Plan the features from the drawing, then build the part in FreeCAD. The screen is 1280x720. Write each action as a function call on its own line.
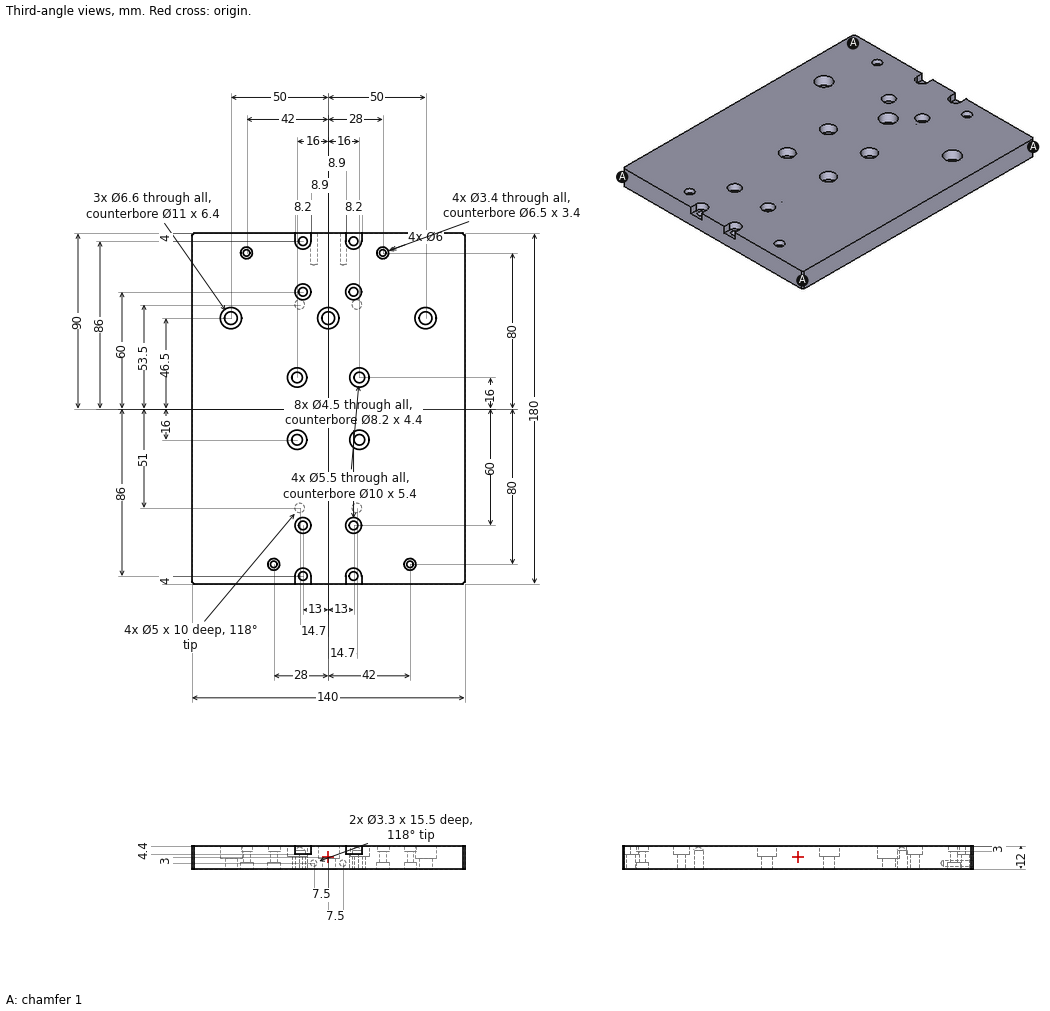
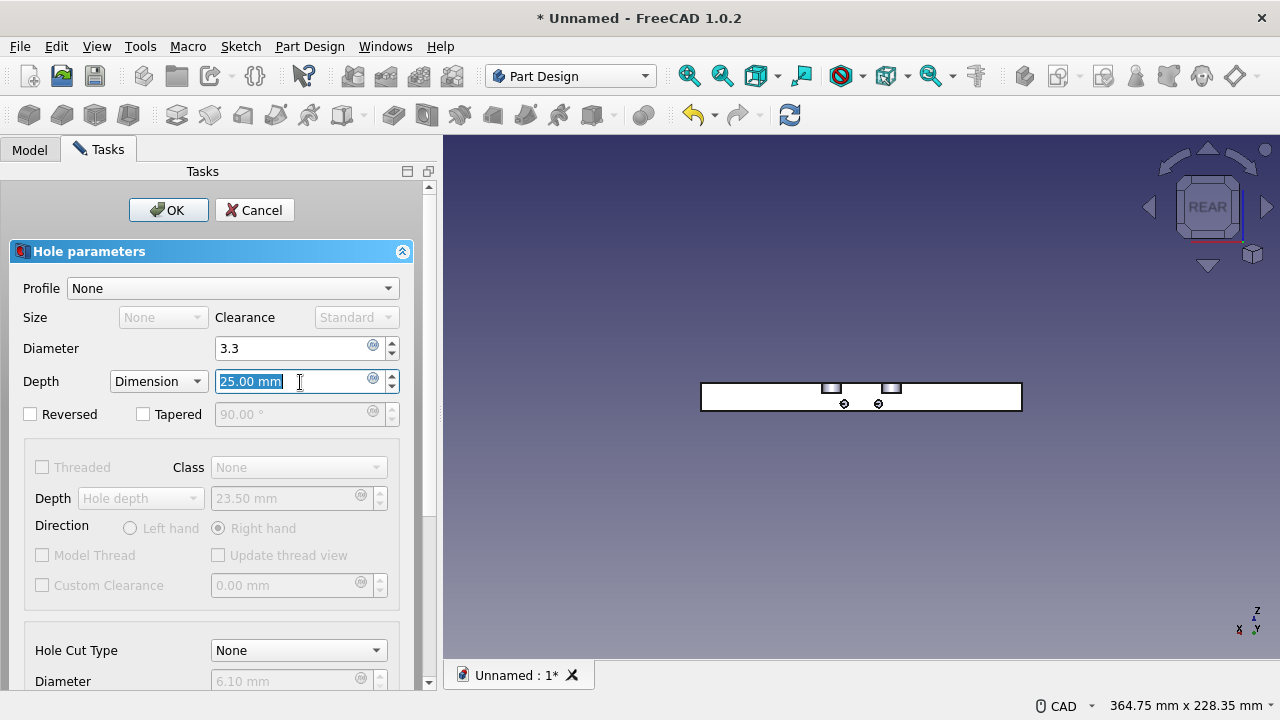
text(15.5)
key(Tab)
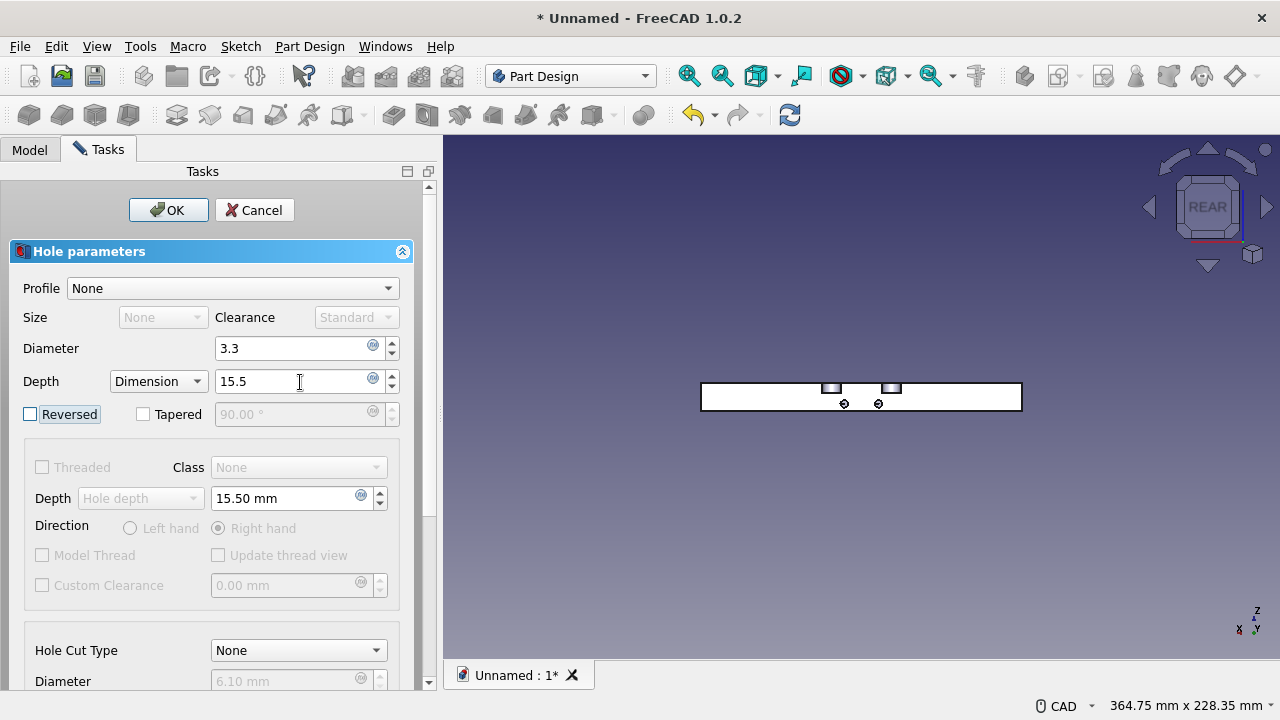
click(169, 210)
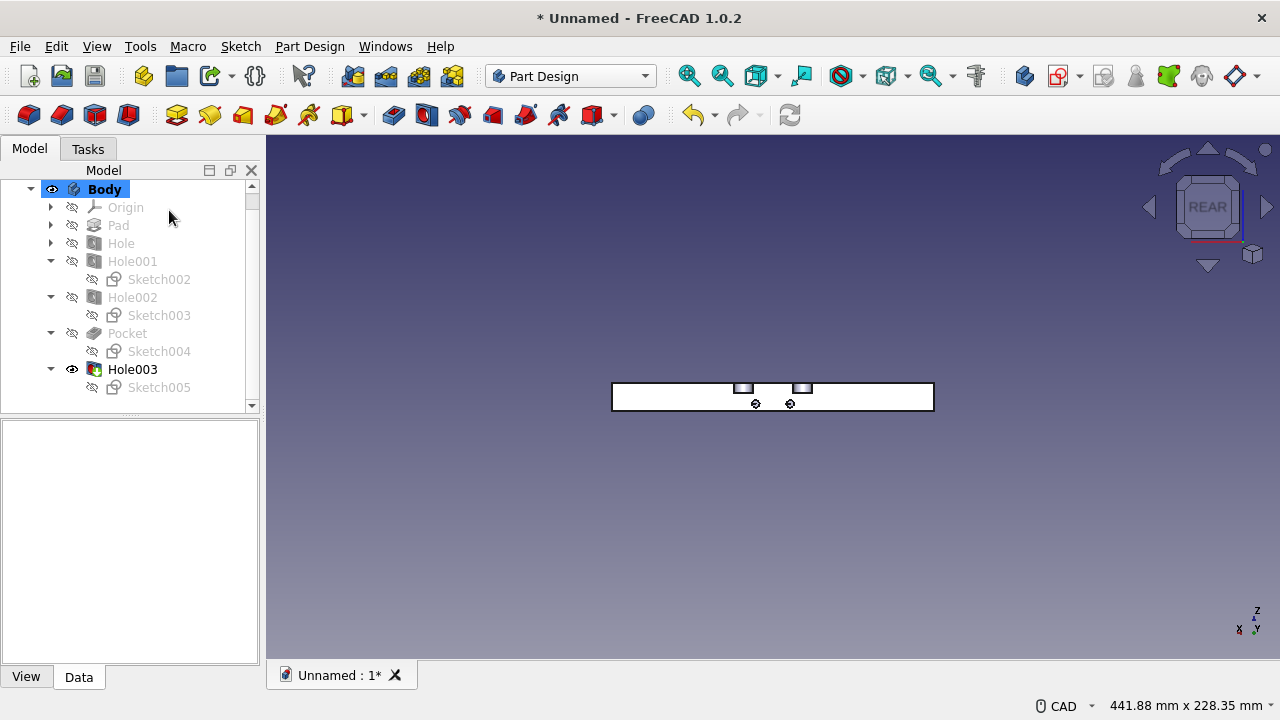
click(690, 76)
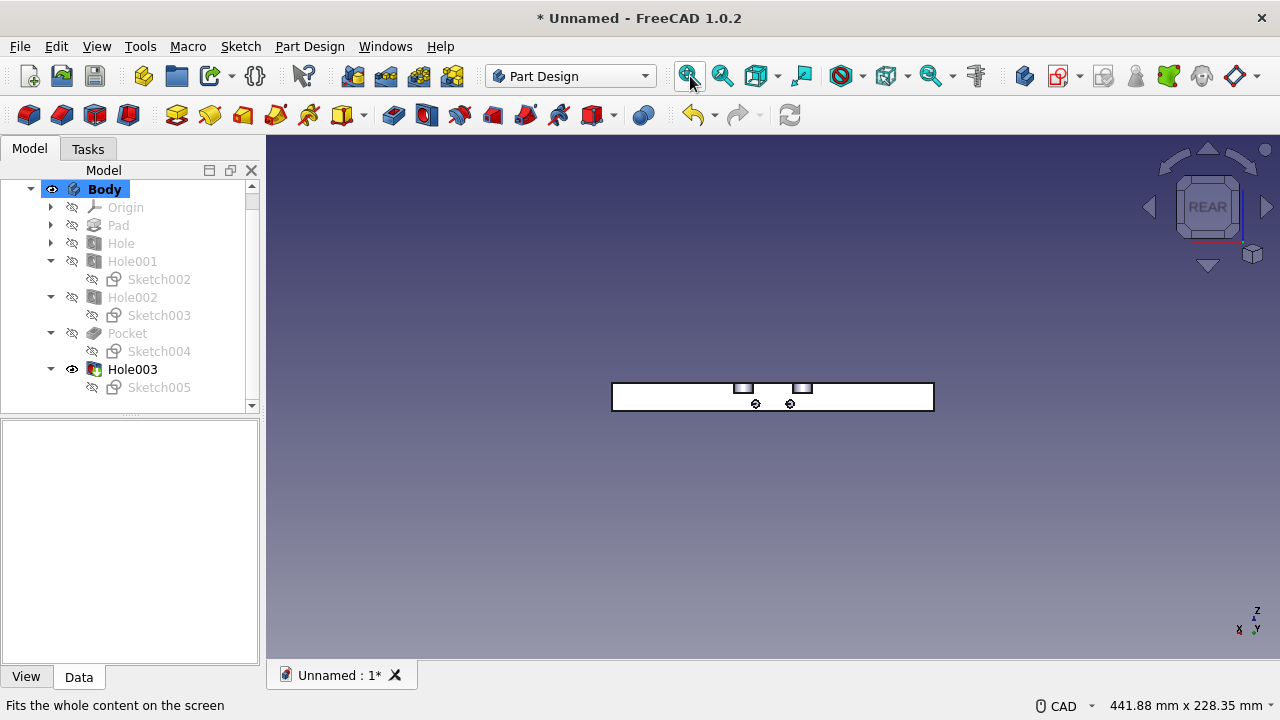
key(0)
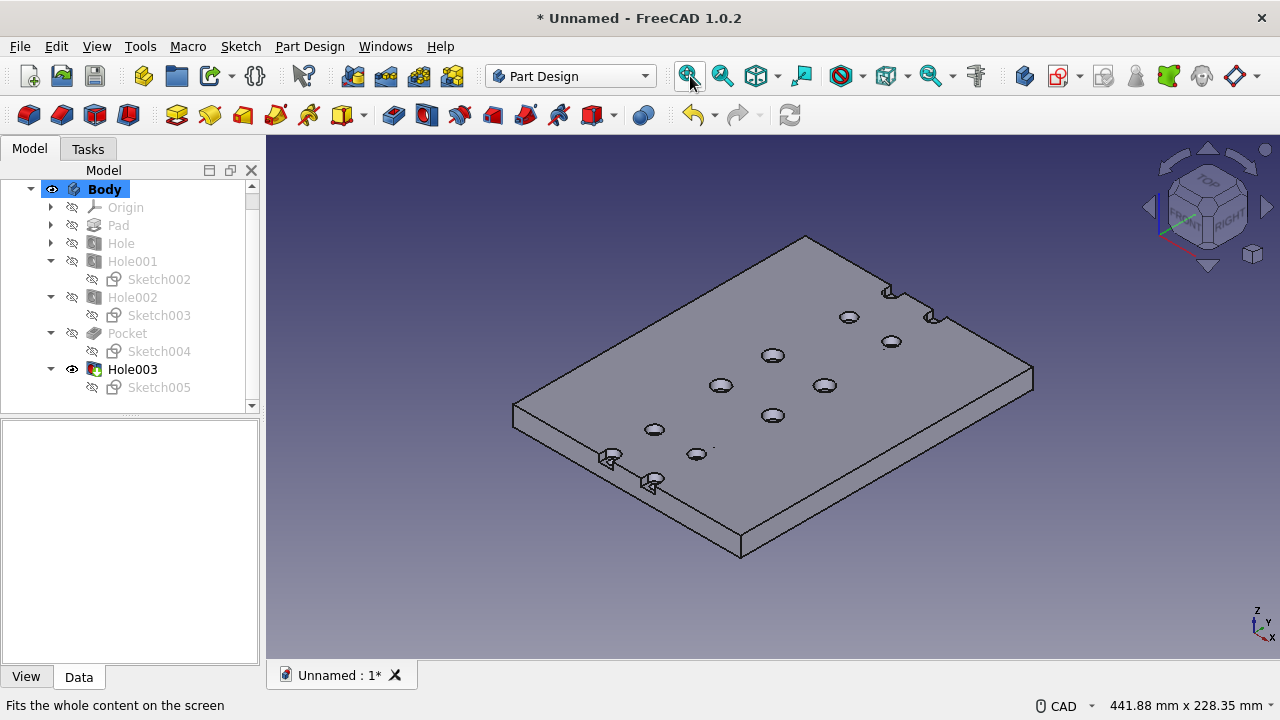
click(921, 374)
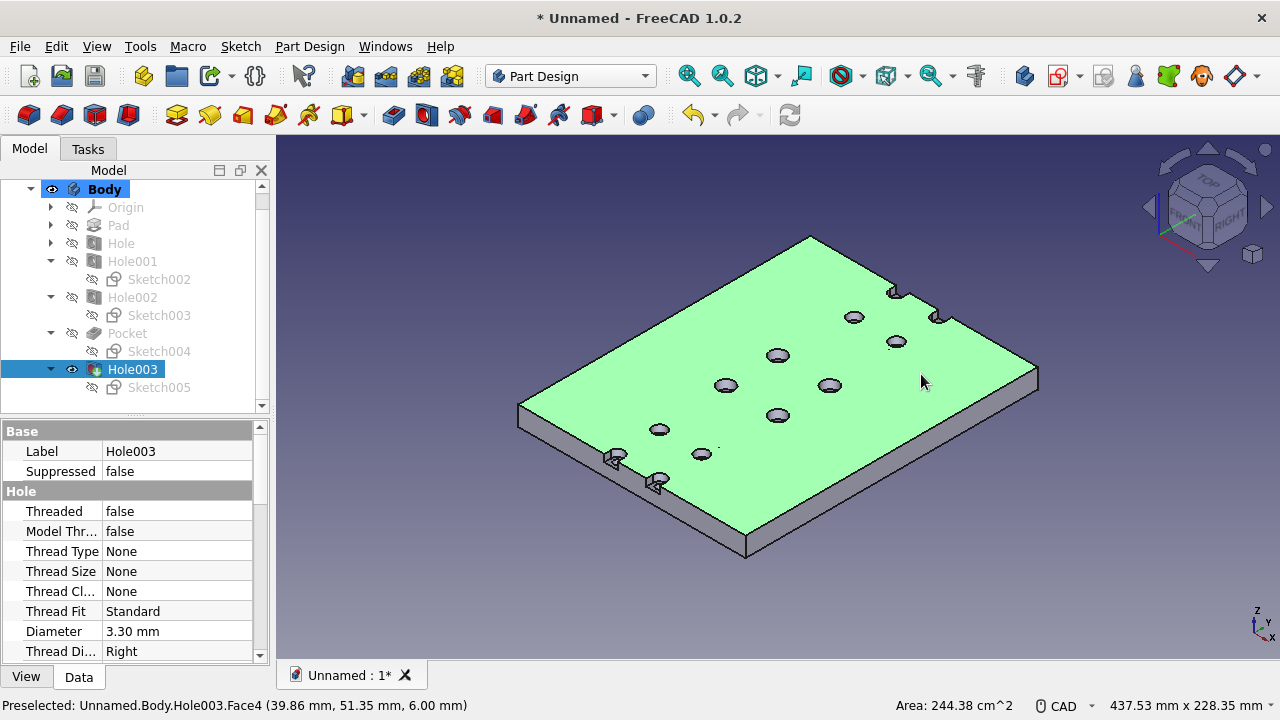
click(1058, 76)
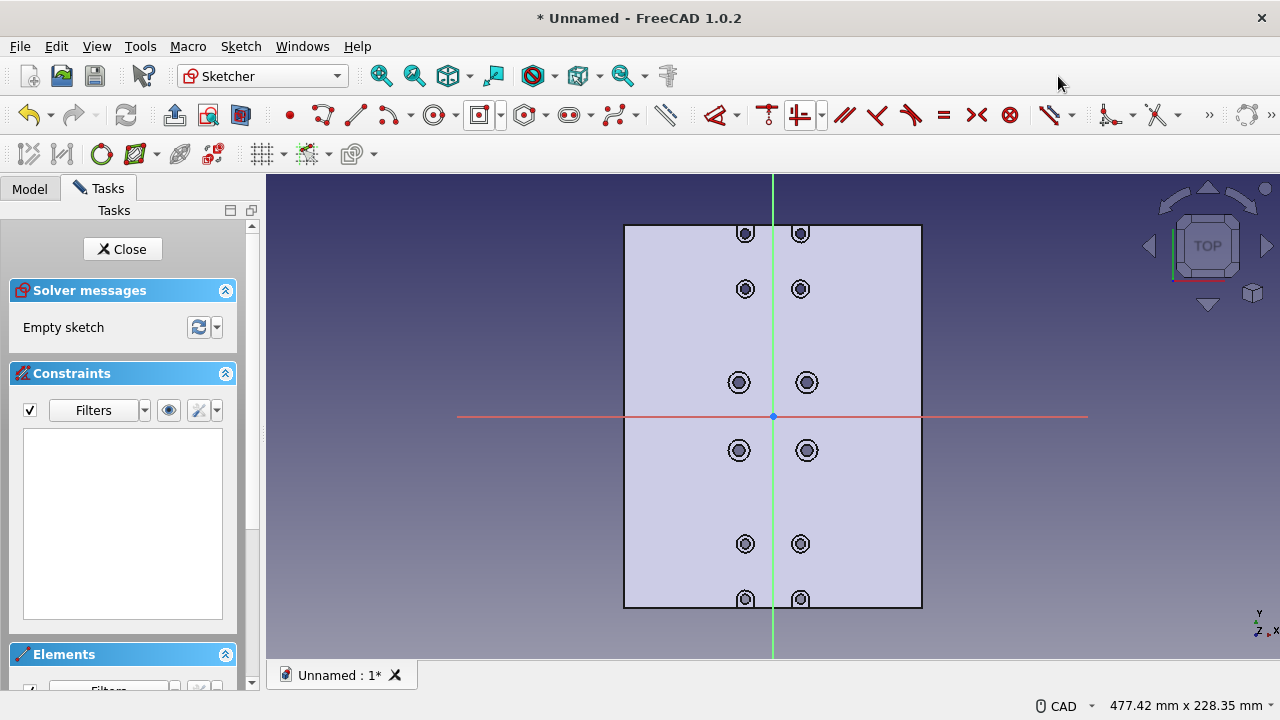
click(434, 116)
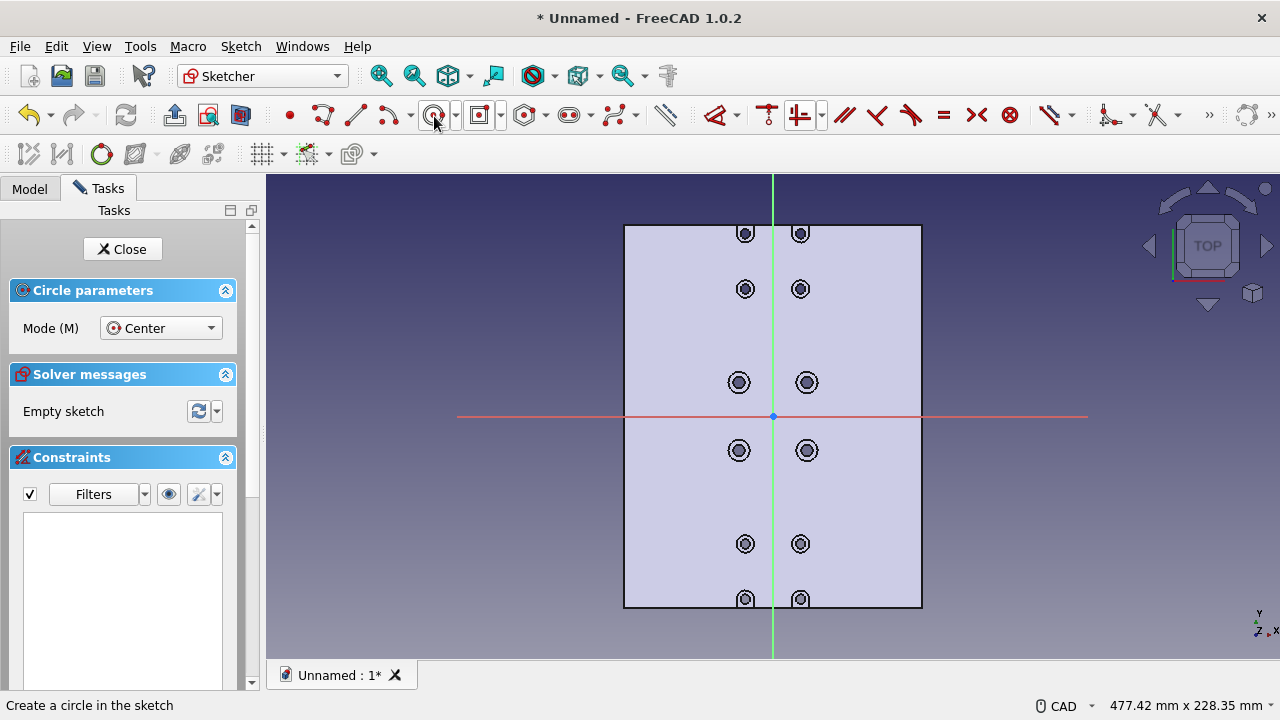
scroll(832, 247, up, 7)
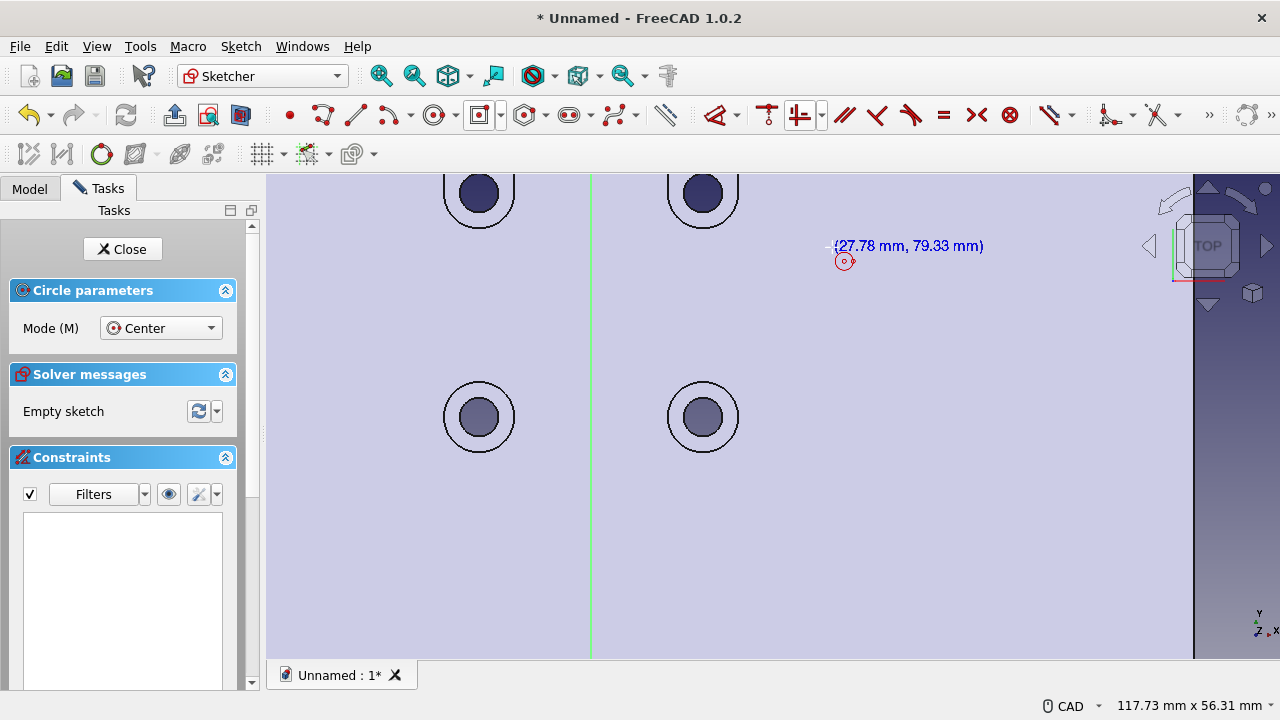
scroll(733, 286, down, 8)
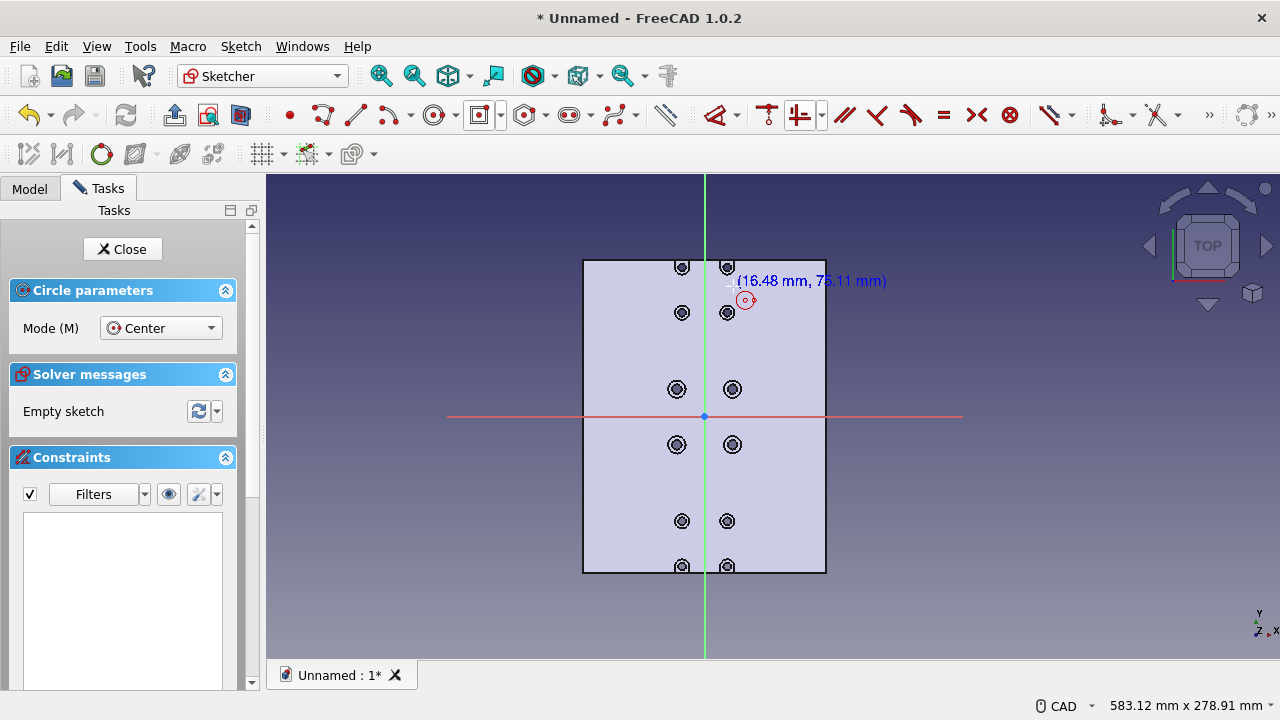
click(753, 278)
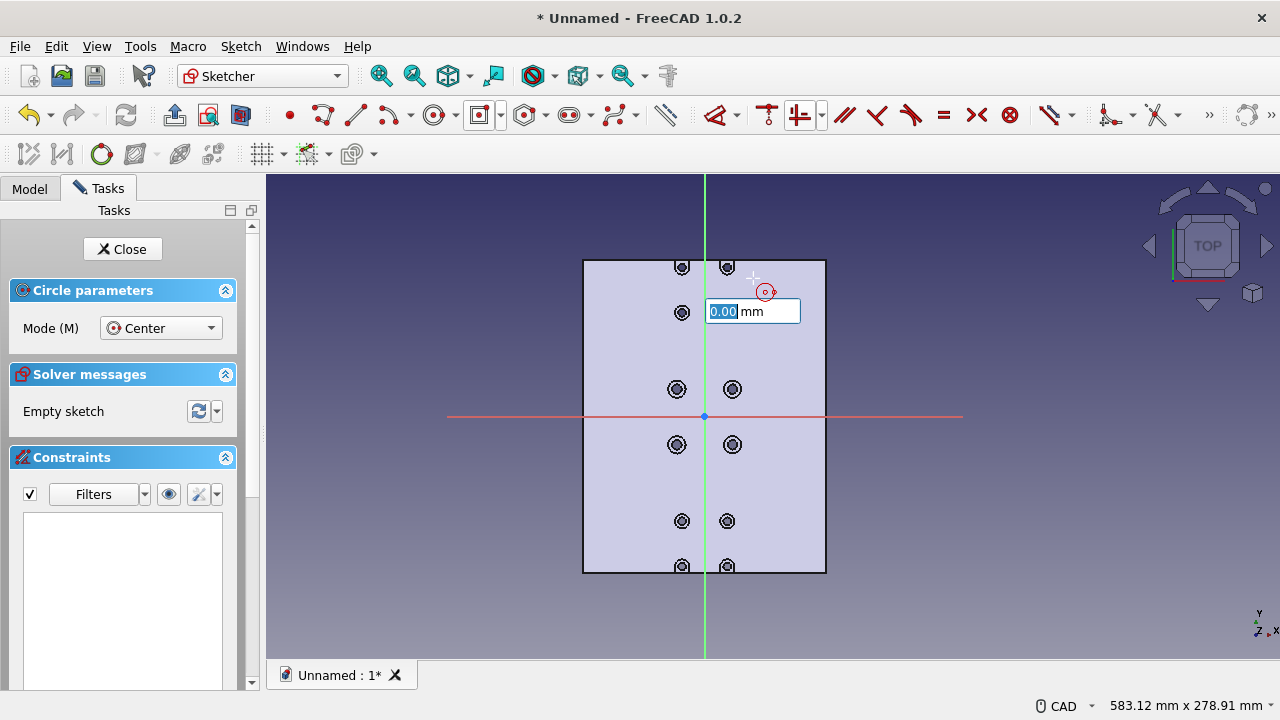
scroll(757, 274, up, 6)